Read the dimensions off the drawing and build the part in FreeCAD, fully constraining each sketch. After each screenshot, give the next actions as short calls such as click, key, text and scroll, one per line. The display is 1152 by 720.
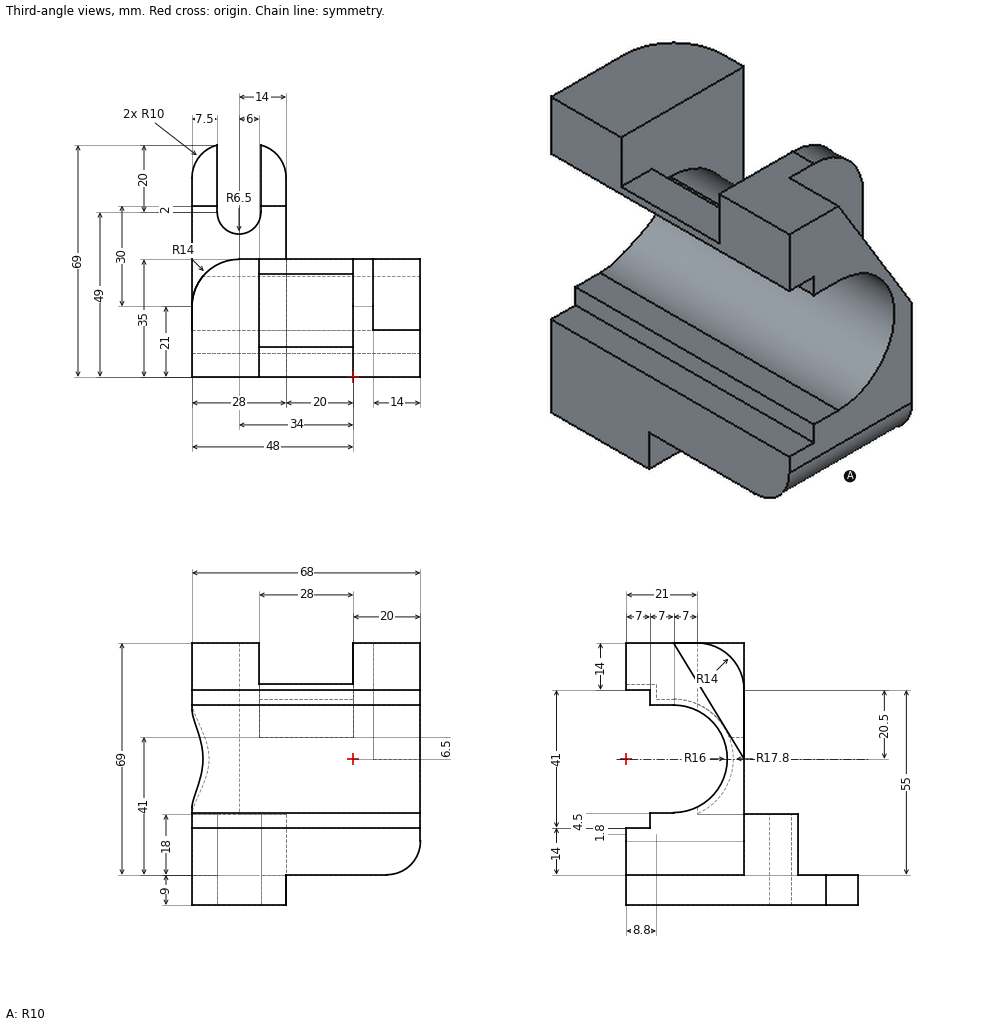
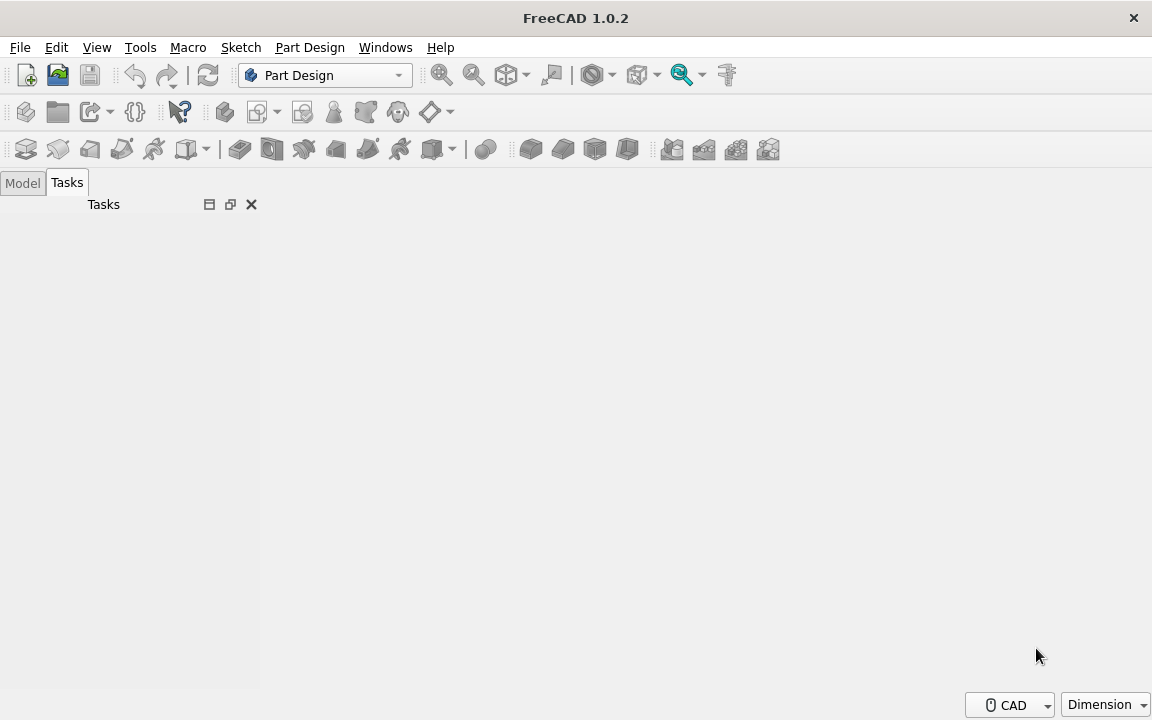
click(26, 76)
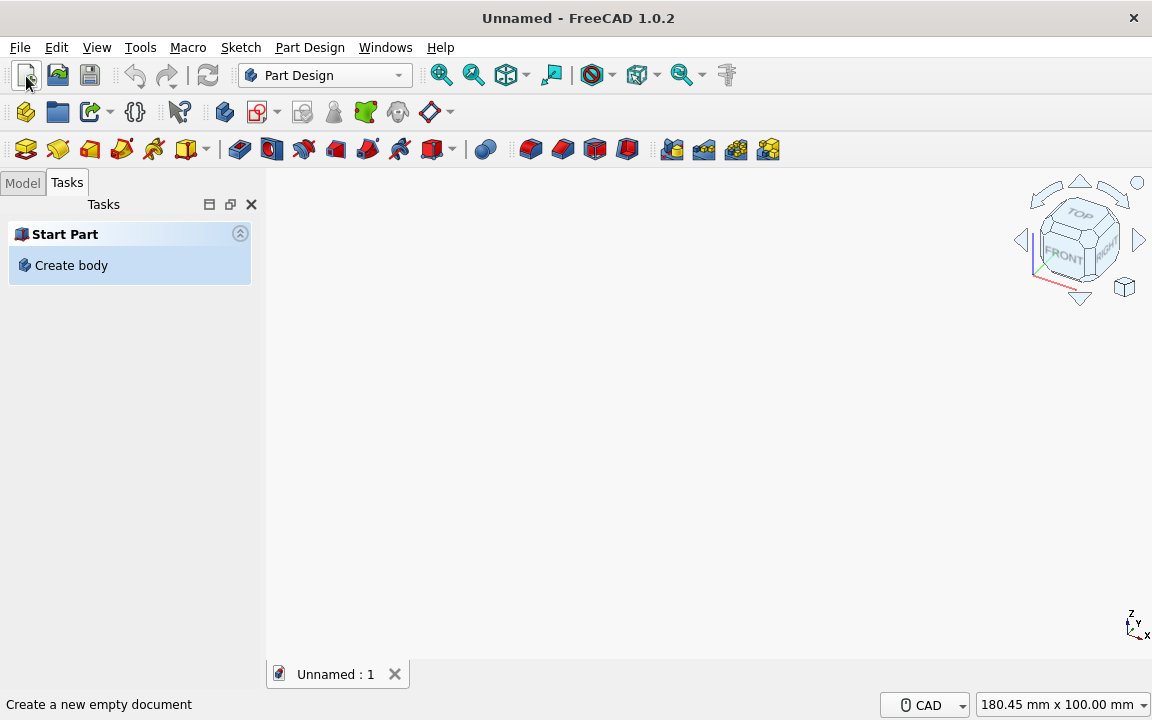
click(258, 112)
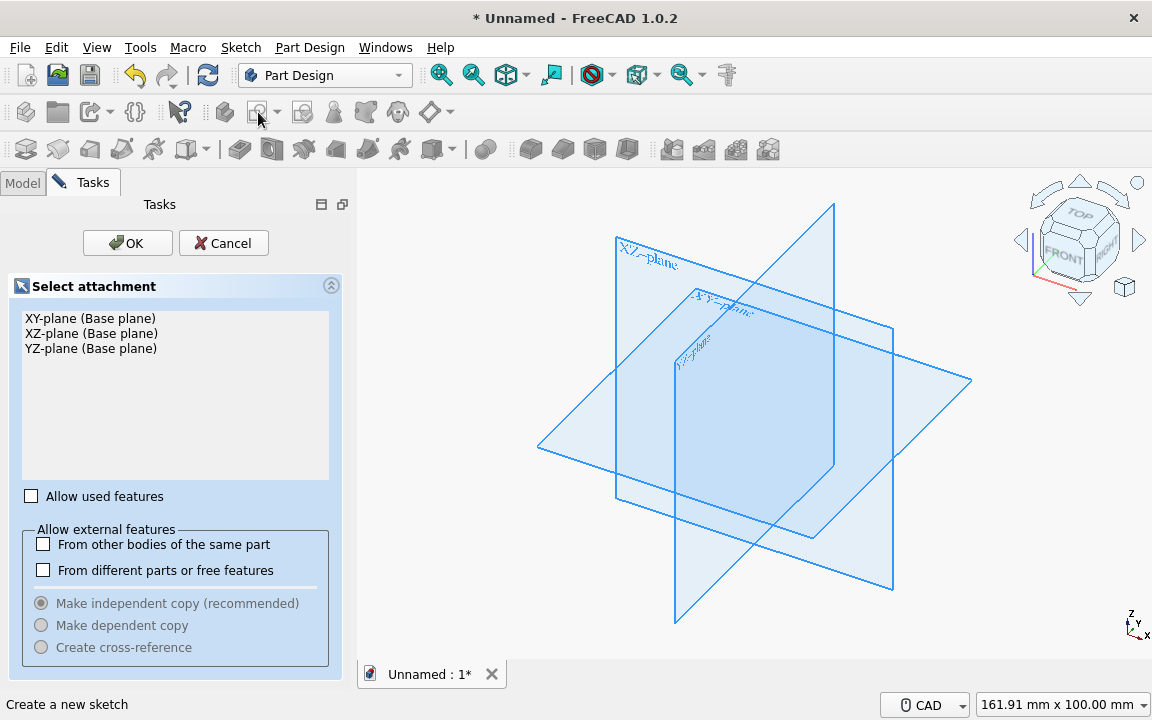
click(82, 348)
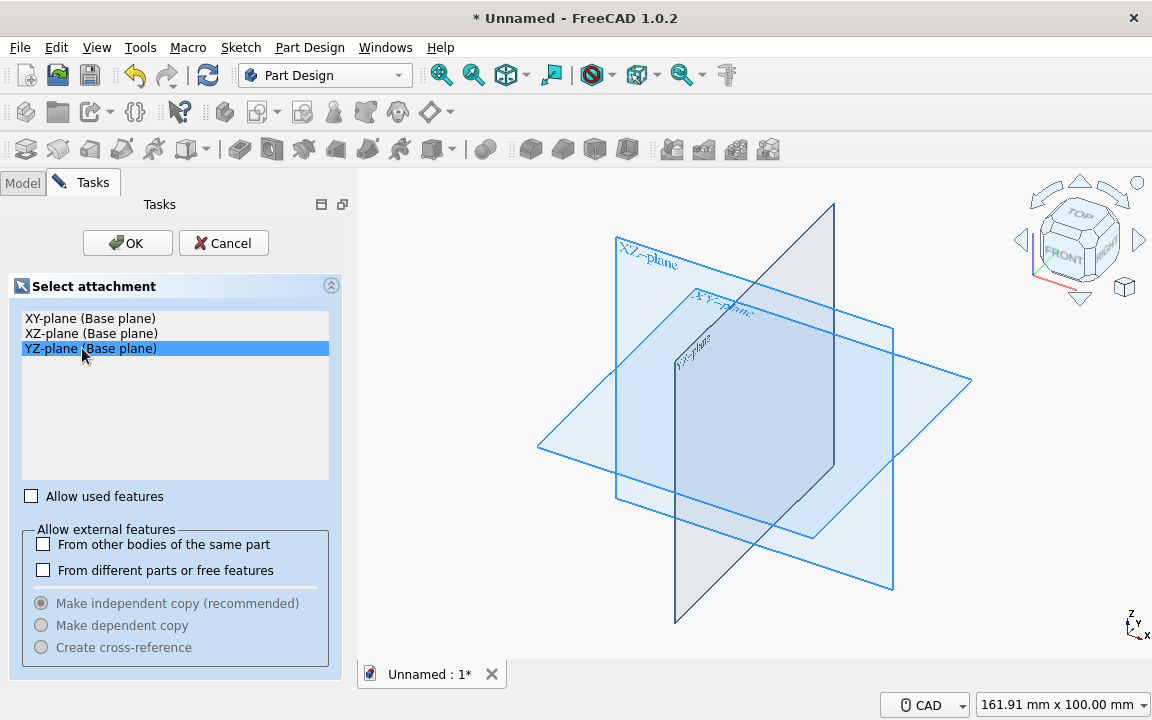
click(128, 243)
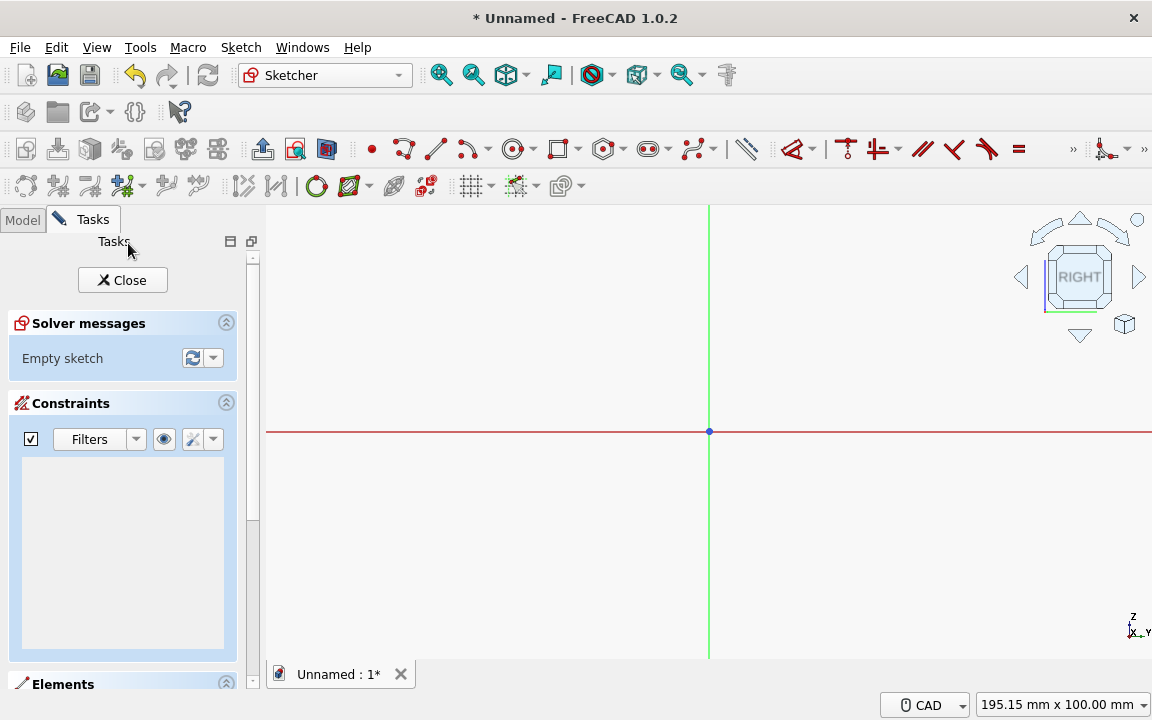
click(404, 150)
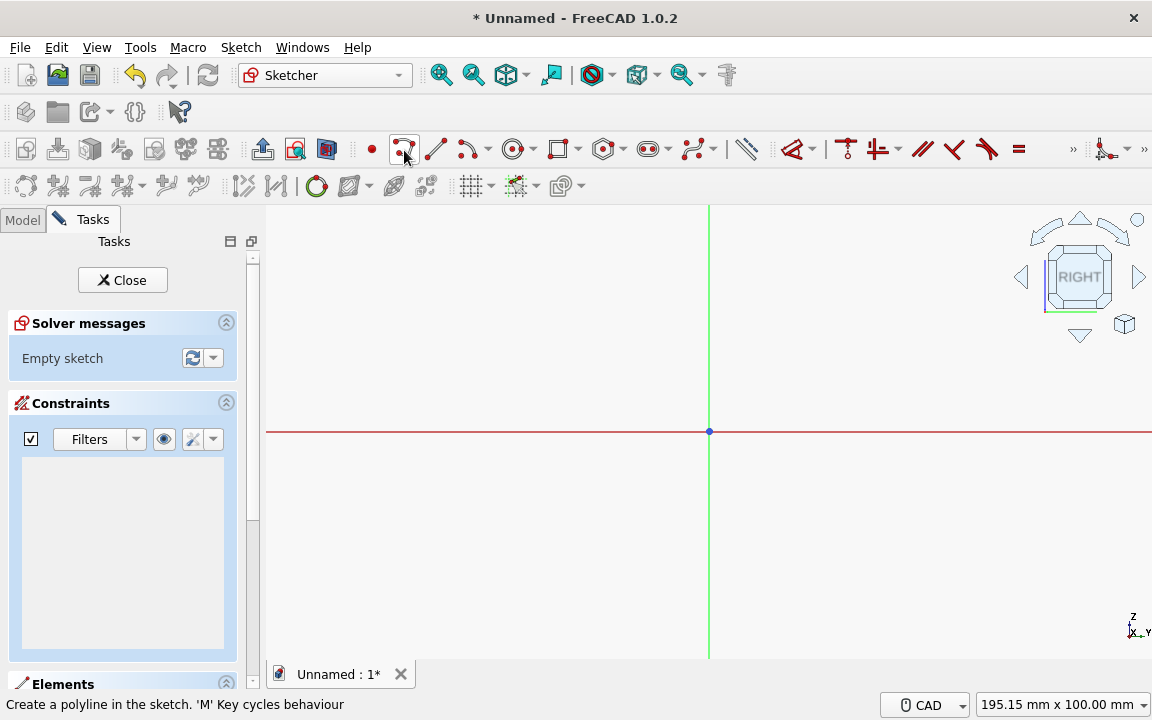
click(804, 275)
click(709, 275)
click(718, 339)
click(741, 339)
click(741, 359)
click(773, 359)
right_click(773, 359)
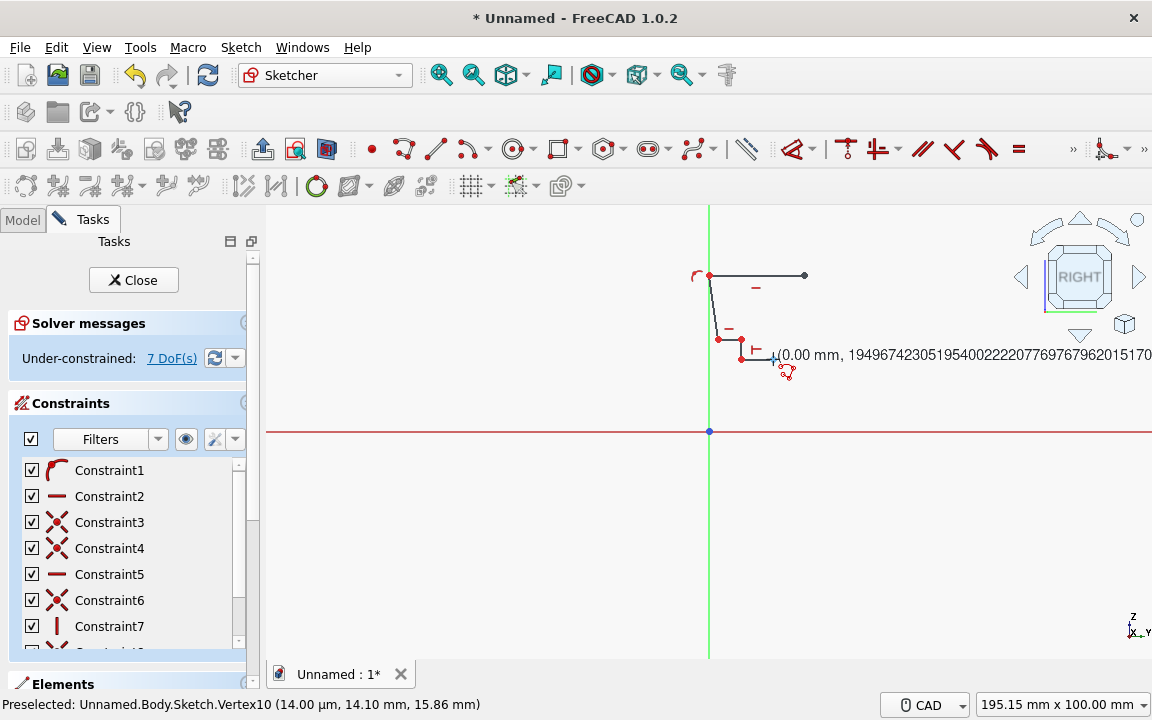
click(773, 505)
click(741, 505)
click(741, 525)
click(709, 525)
click(718, 589)
click(868, 589)
click(868, 339)
right_click(868, 339)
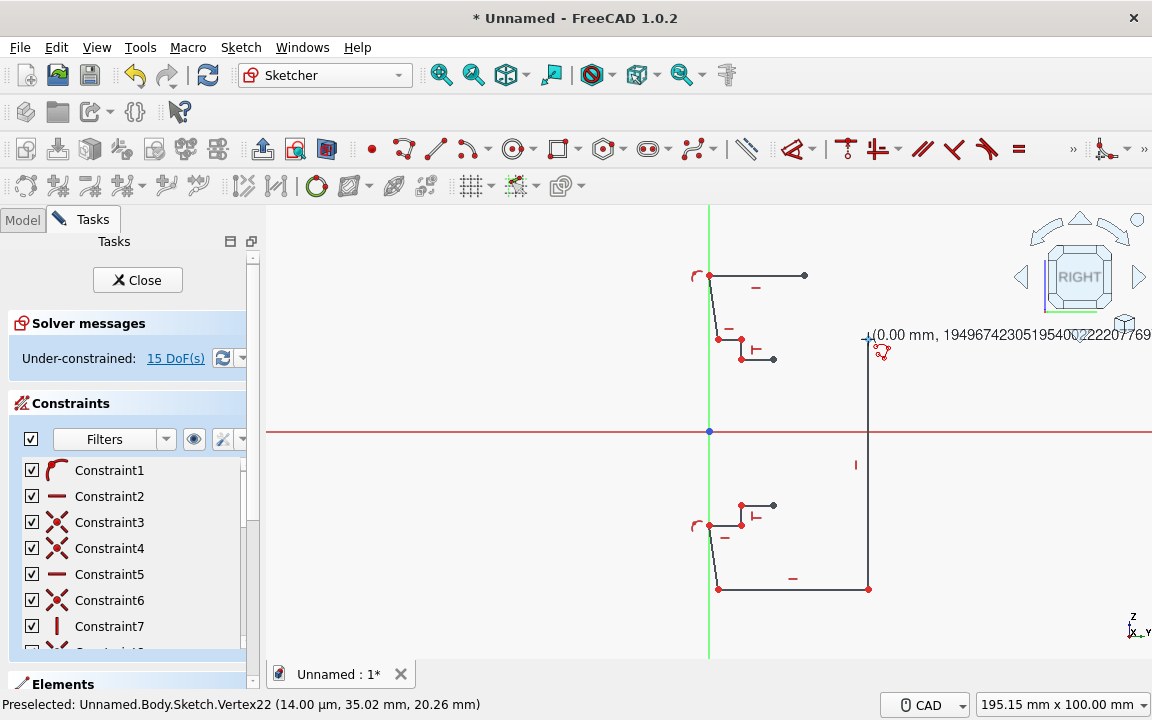
click(490, 150)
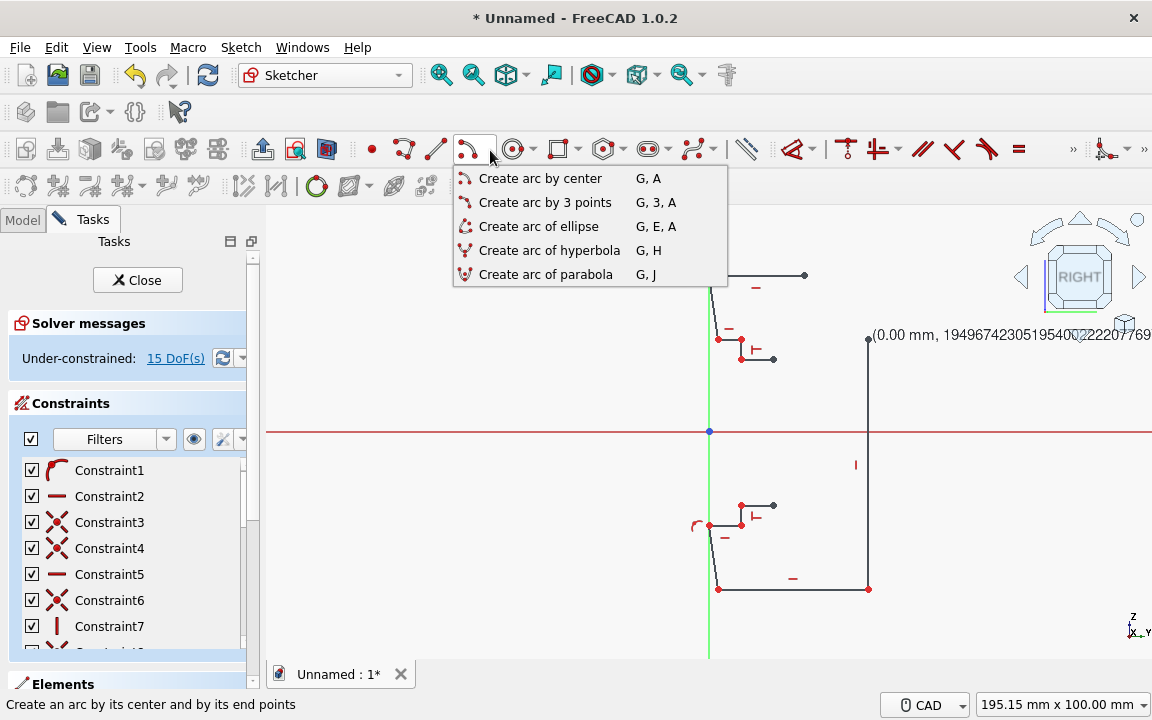
click(590, 202)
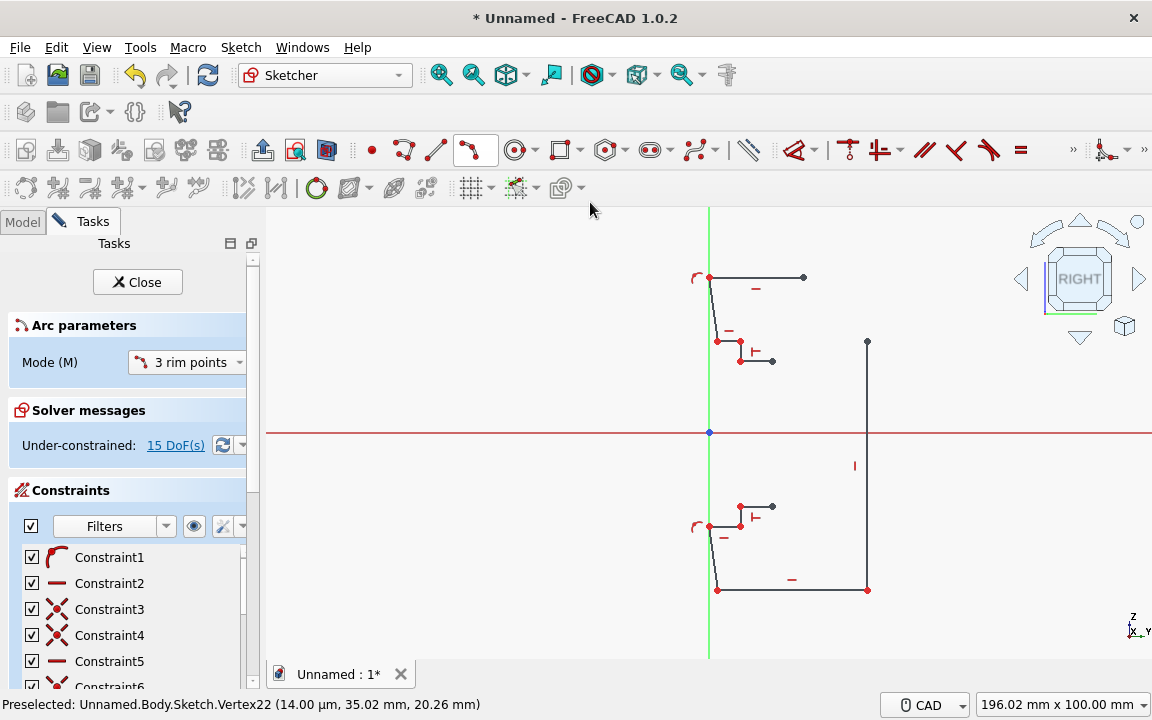
click(773, 361)
click(773, 507)
click(841, 455)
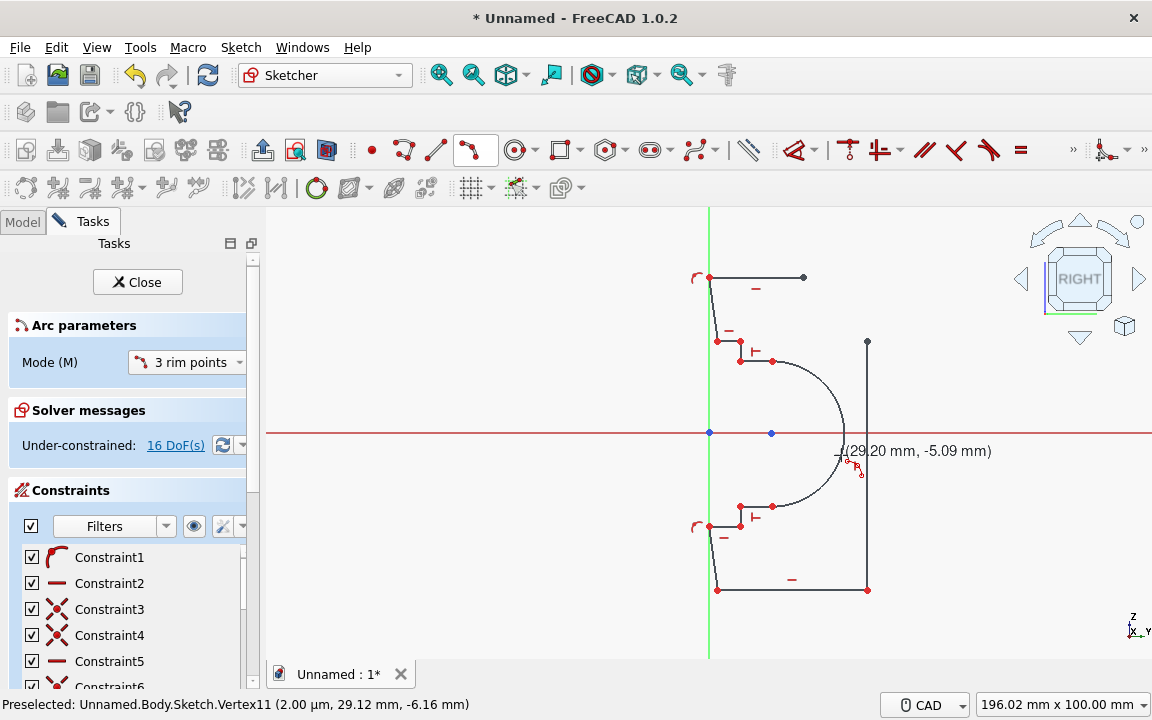
click(867, 341)
click(804, 278)
click(849, 296)
key(Escape)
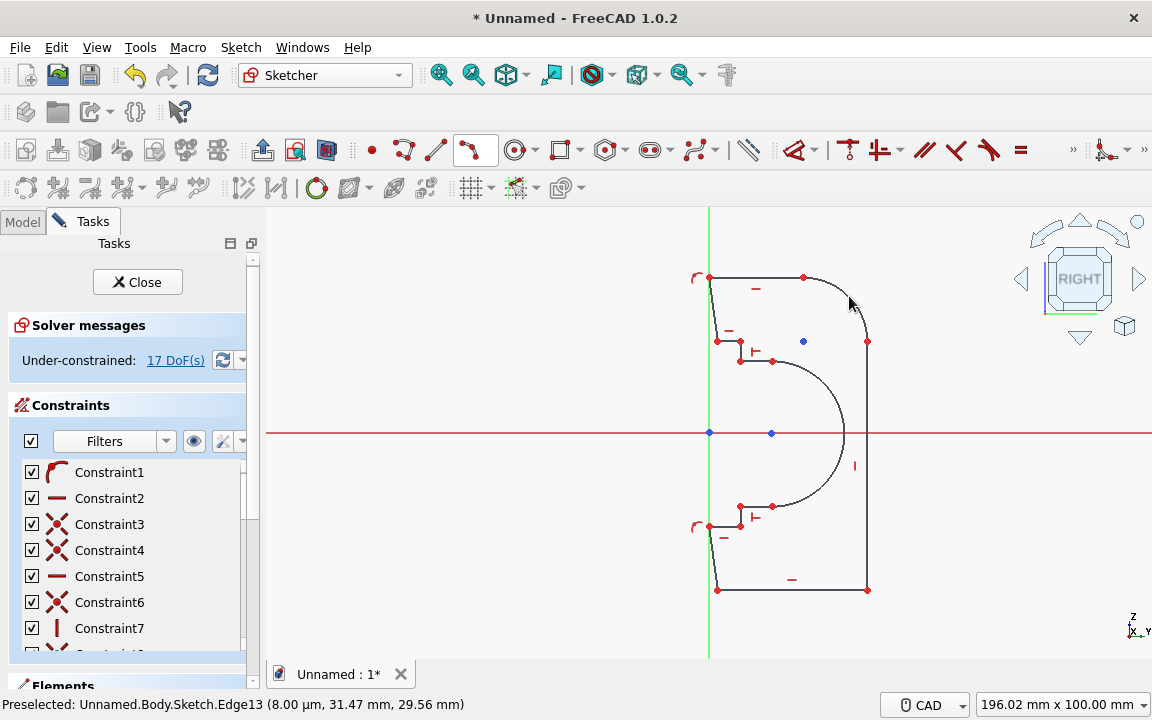
click(775, 278)